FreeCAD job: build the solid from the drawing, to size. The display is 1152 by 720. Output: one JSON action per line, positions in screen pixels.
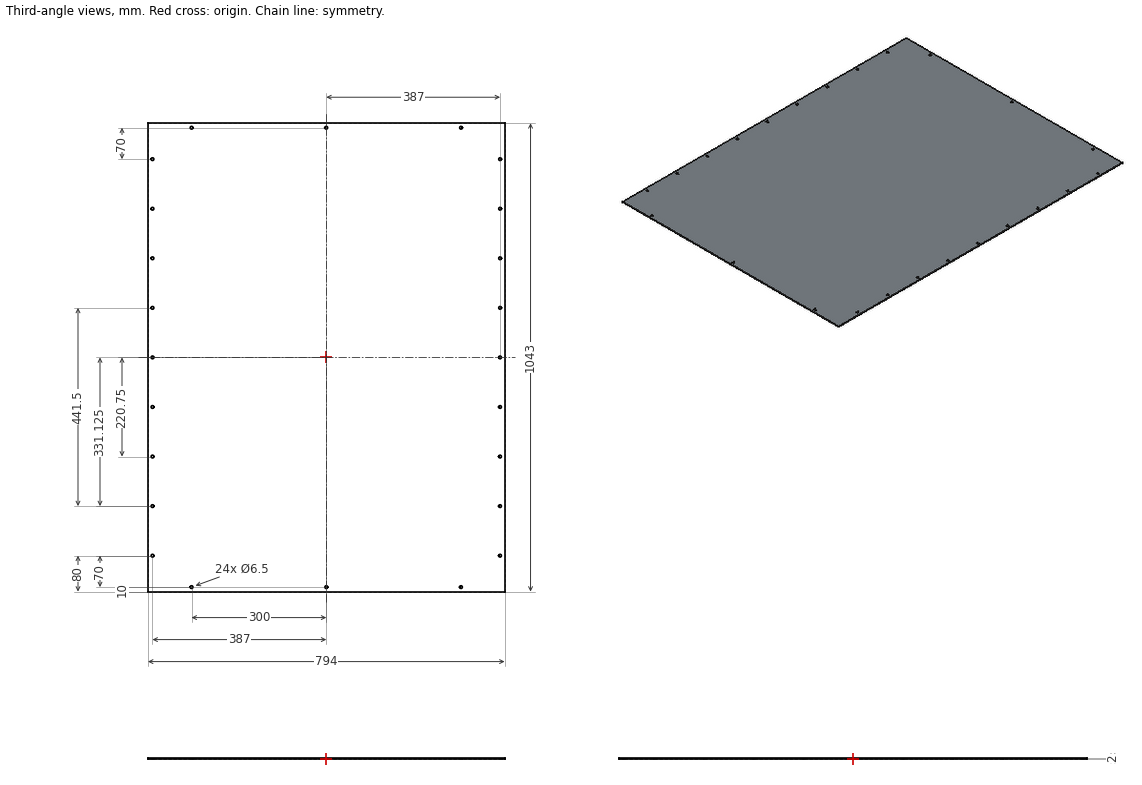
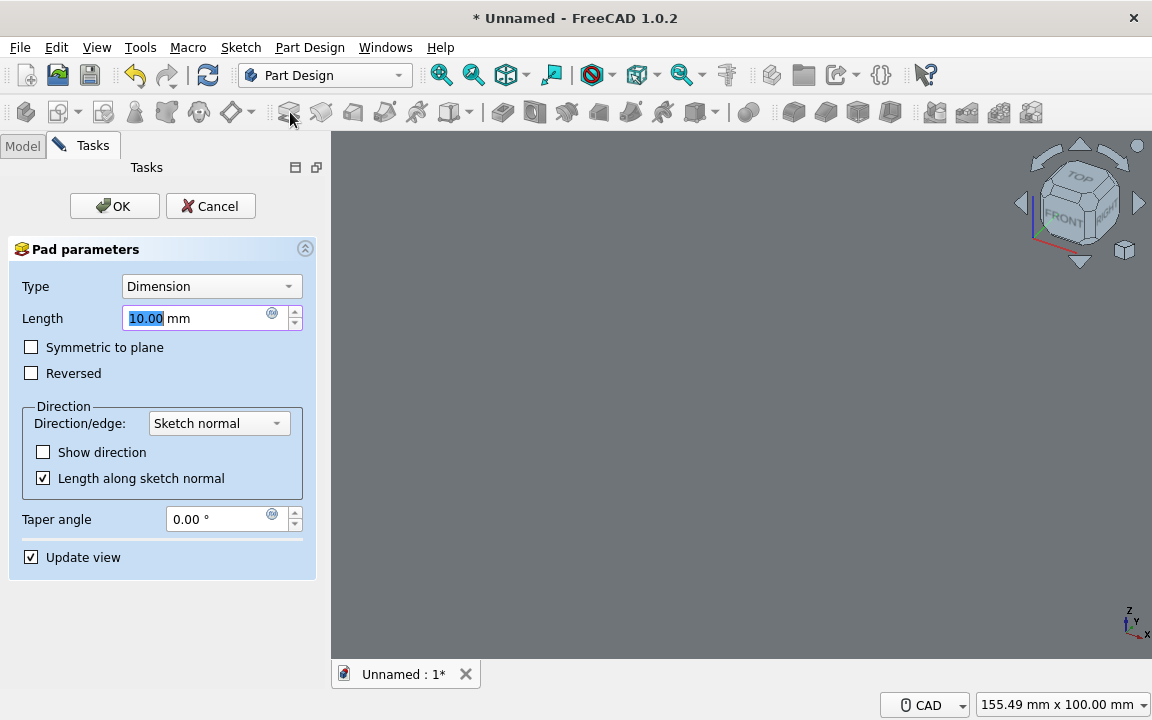
{"action": "type", "text": "2"}
{"action": "key", "text": "Tab"}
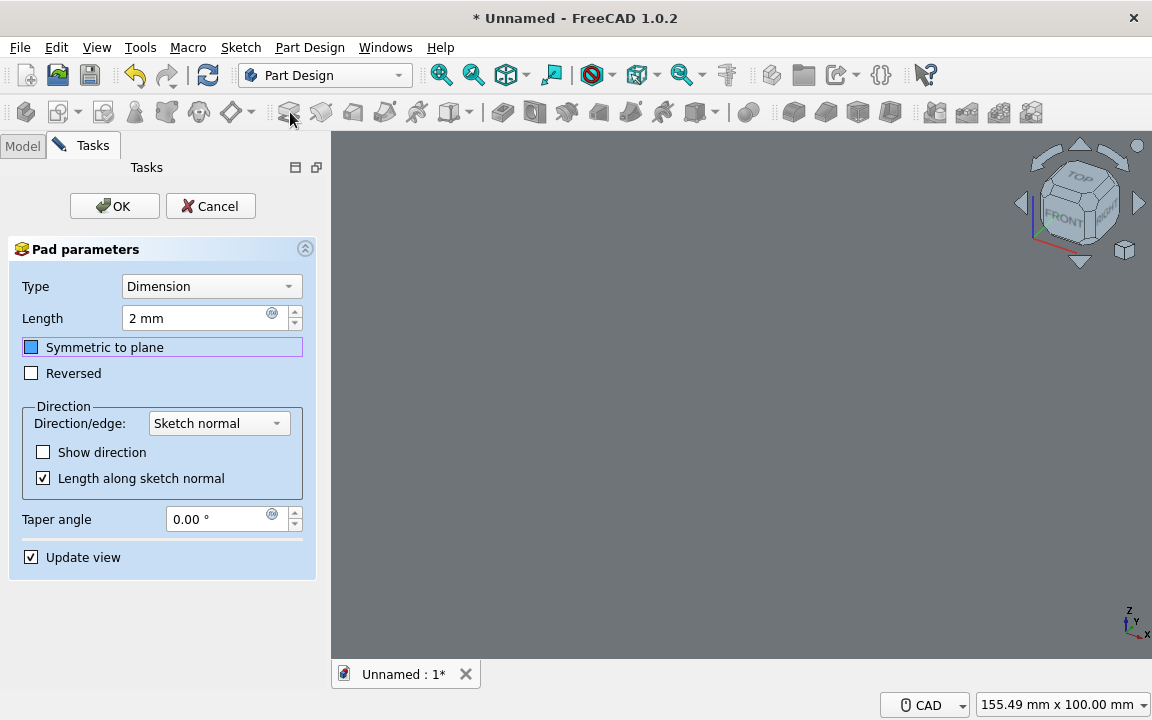
{"action": "left_click", "coordinate": [115, 206]}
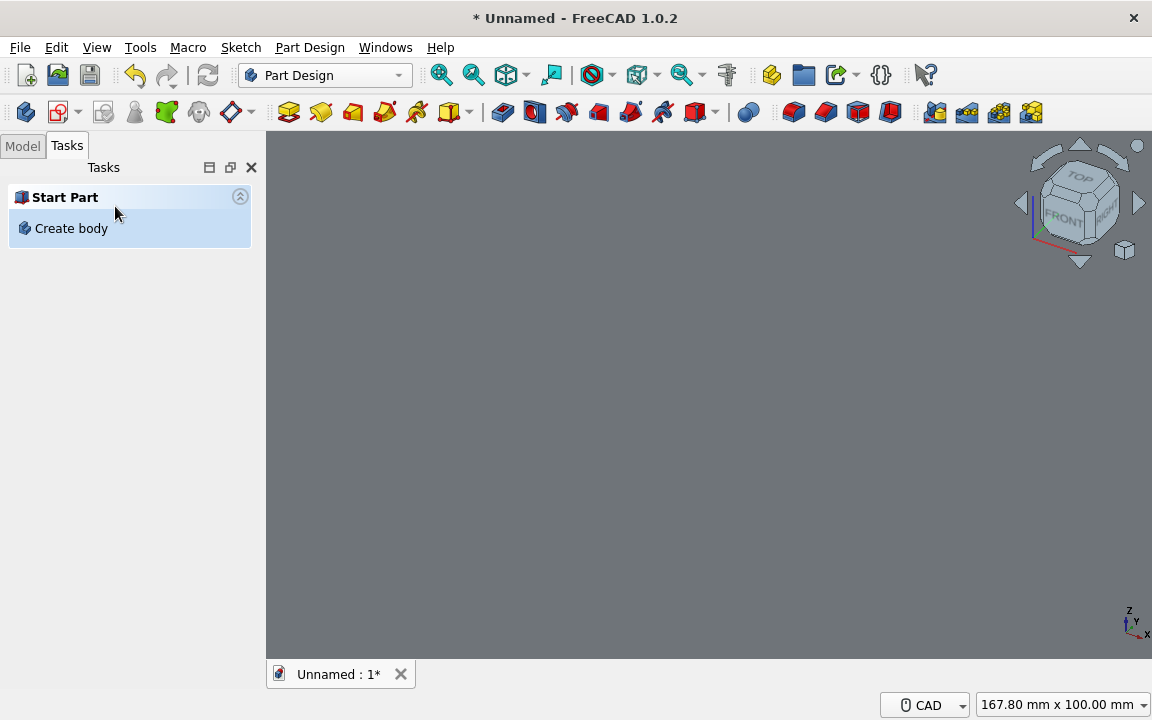
{"action": "key", "text": "0"}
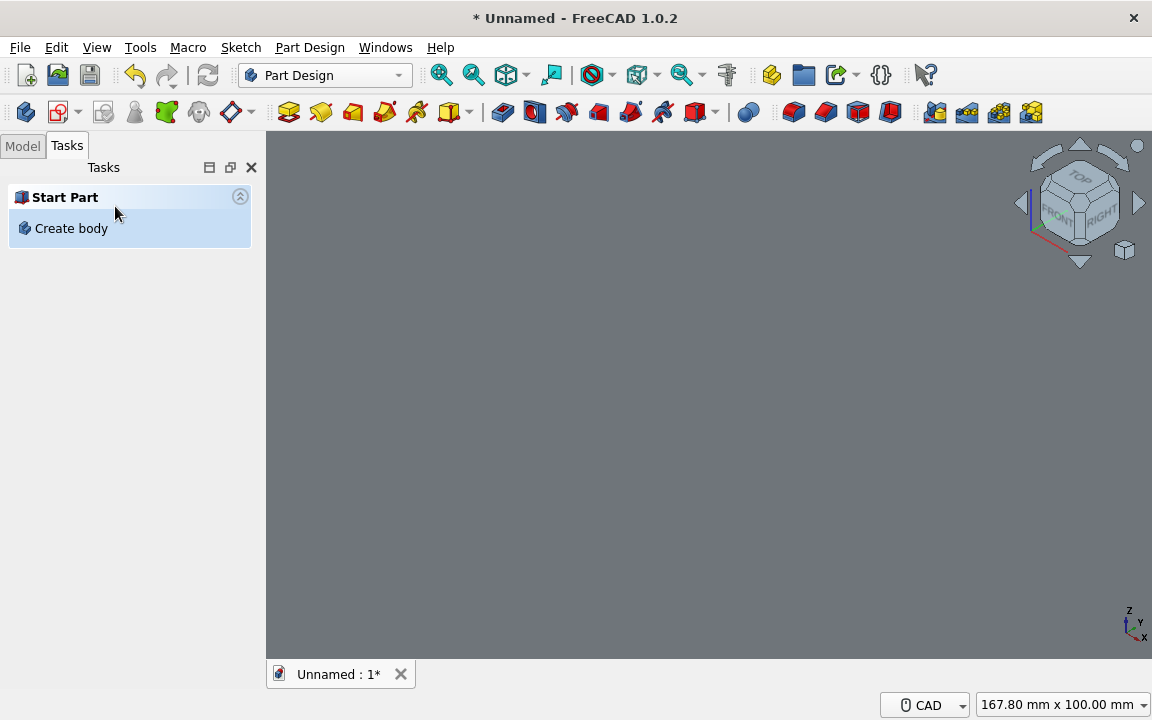
{"action": "left_click", "coordinate": [442, 76]}